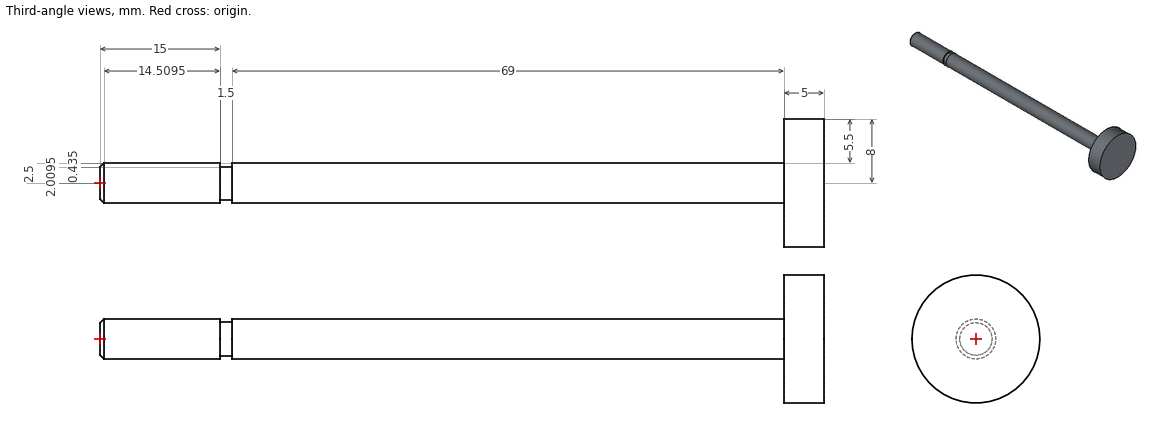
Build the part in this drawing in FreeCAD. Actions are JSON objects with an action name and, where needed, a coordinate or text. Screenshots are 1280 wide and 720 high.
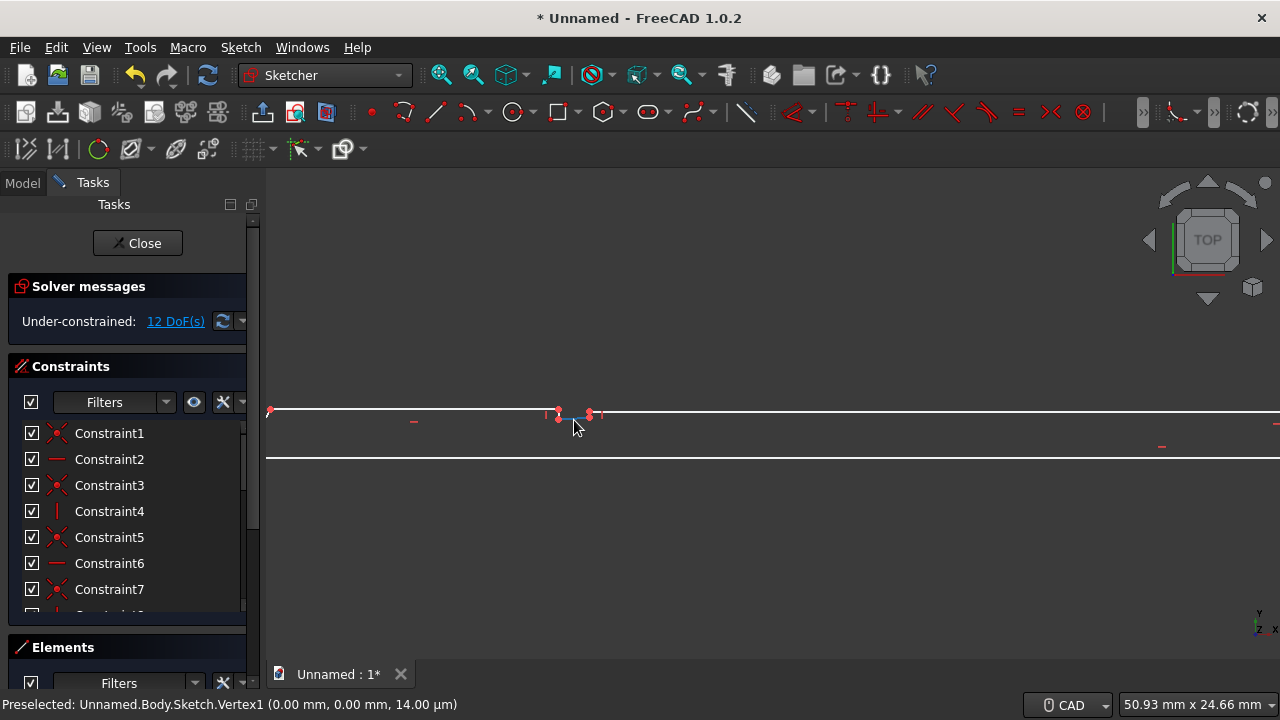
{"action": "left_click", "coordinate": [574, 419]}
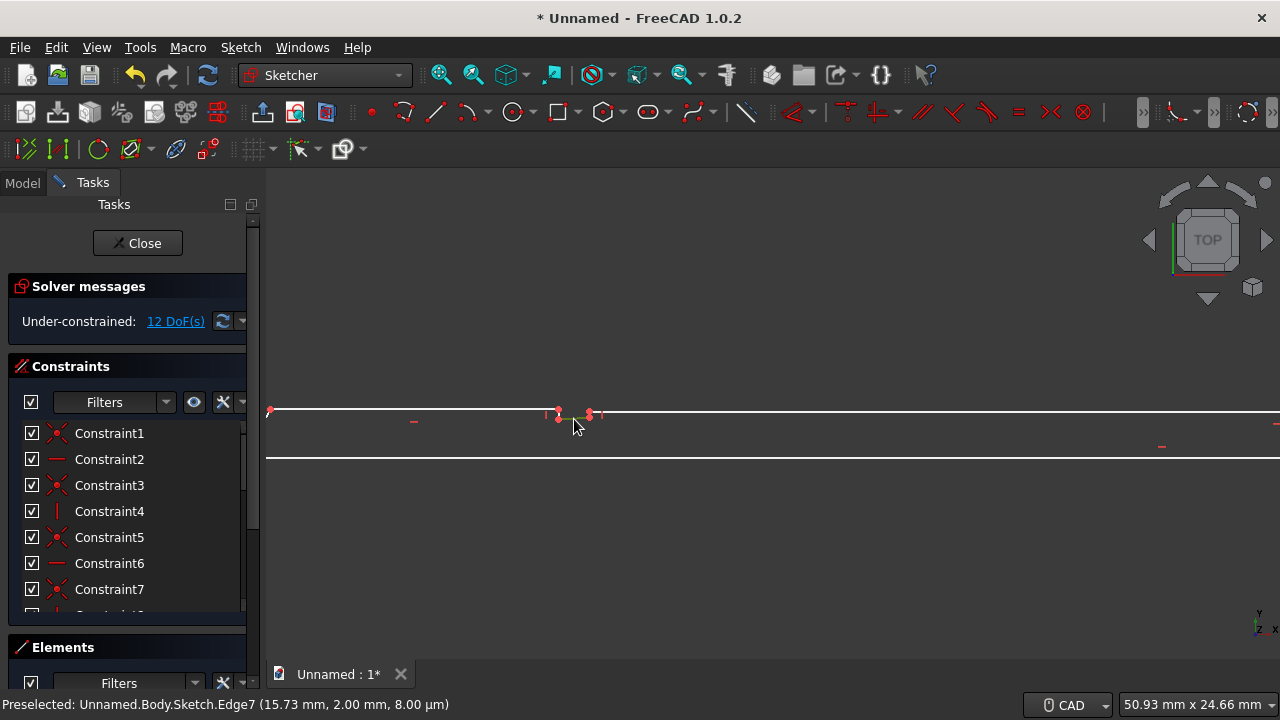
{"action": "key", "text": "h"}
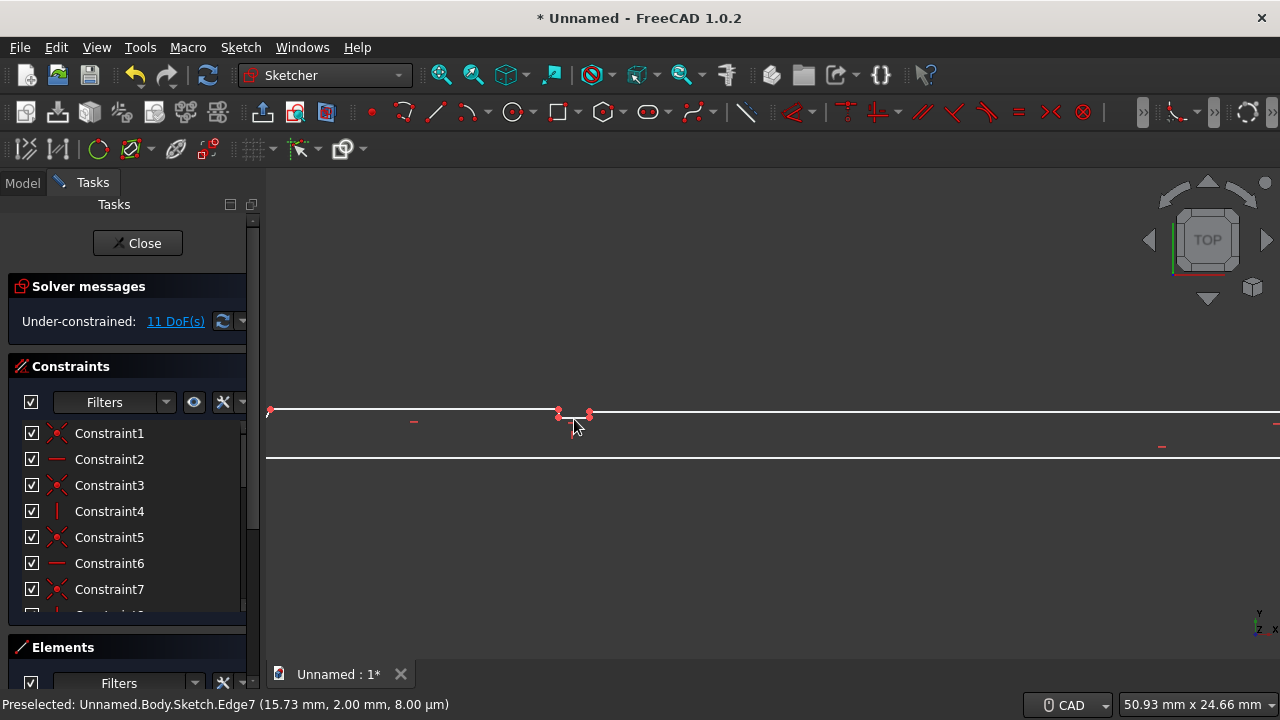
{"action": "scroll", "coordinate": [507, 428], "scroll_direction": "down", "scroll_amount": 6}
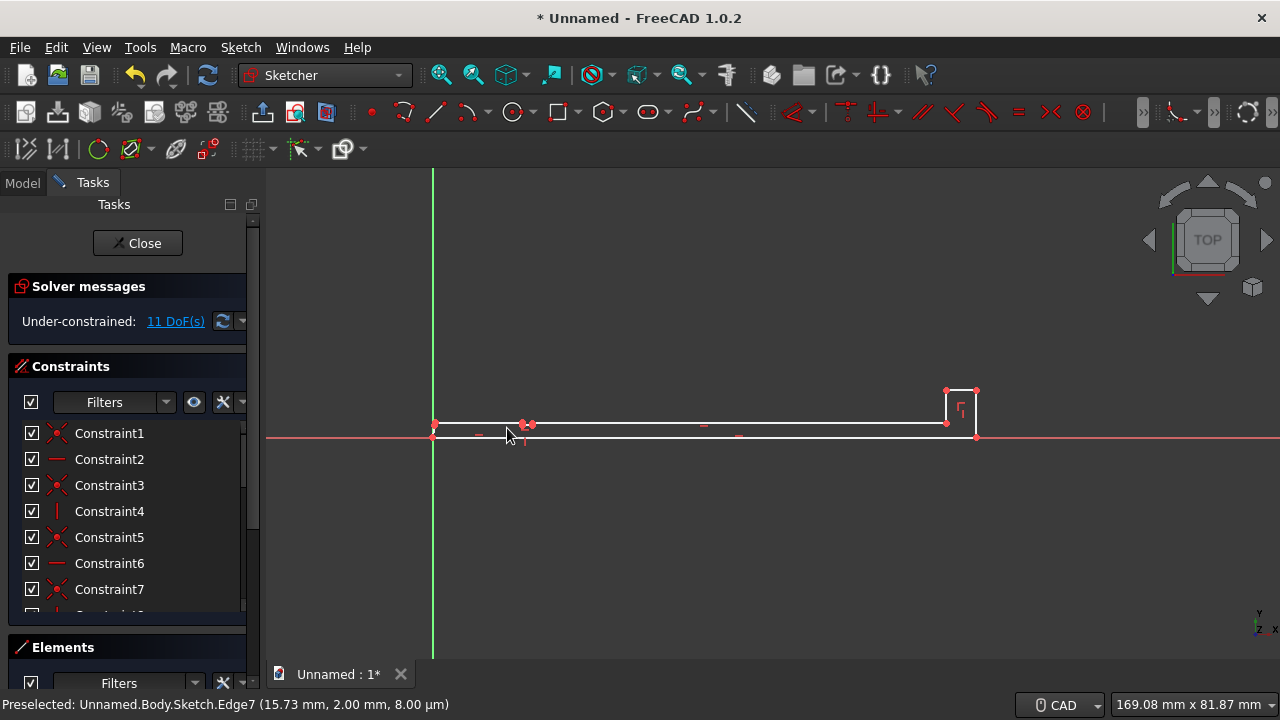
{"action": "scroll", "coordinate": [434, 429], "scroll_direction": "up", "scroll_amount": 7}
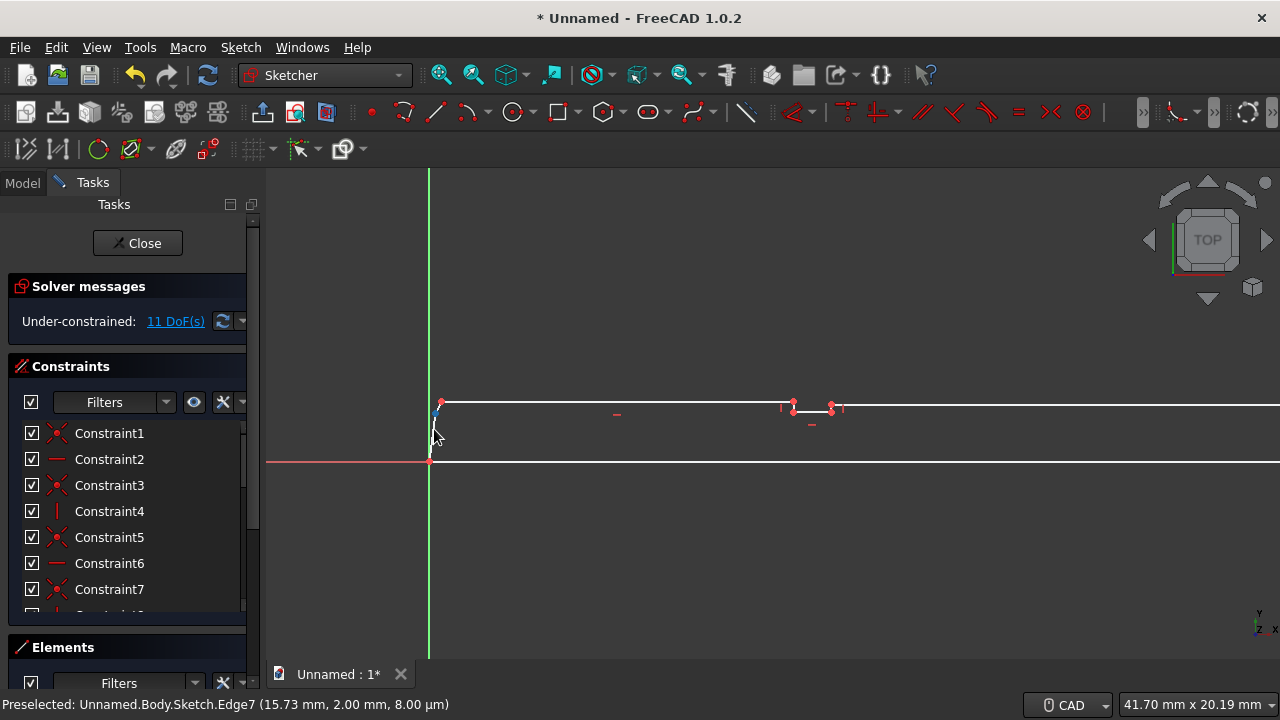
{"action": "left_click", "coordinate": [434, 428]}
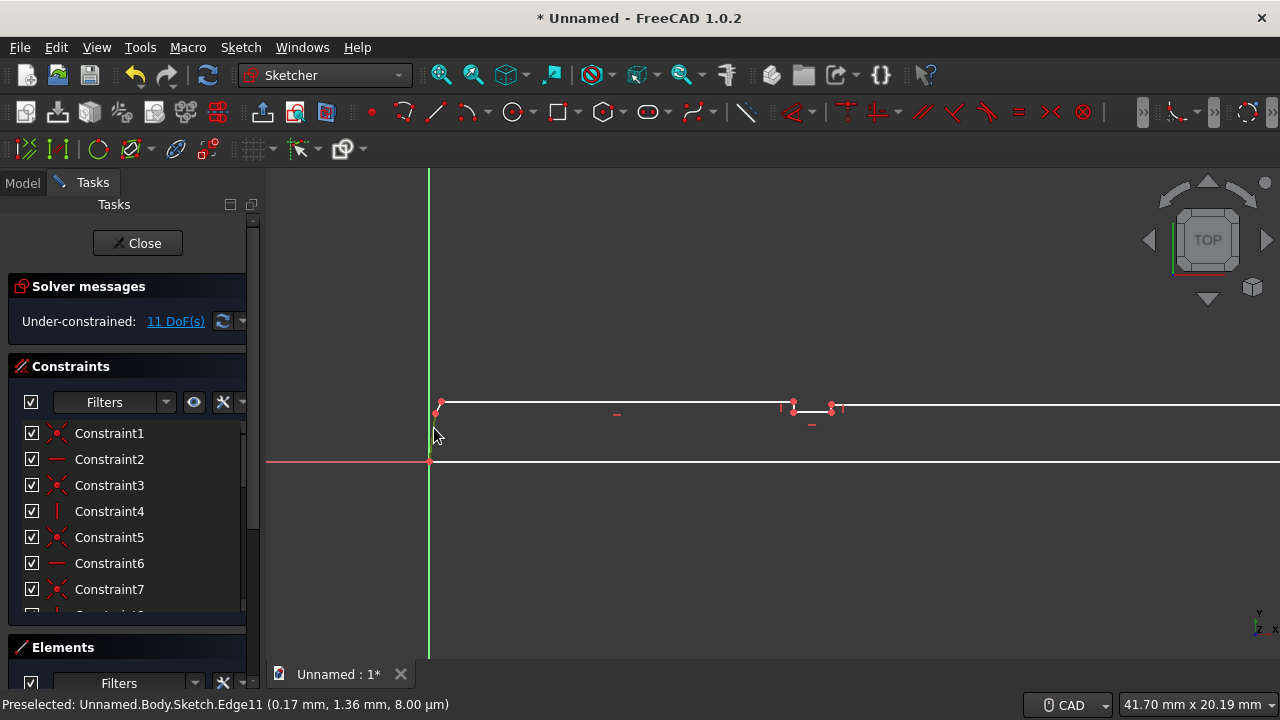
{"action": "left_click", "coordinate": [900, 112]}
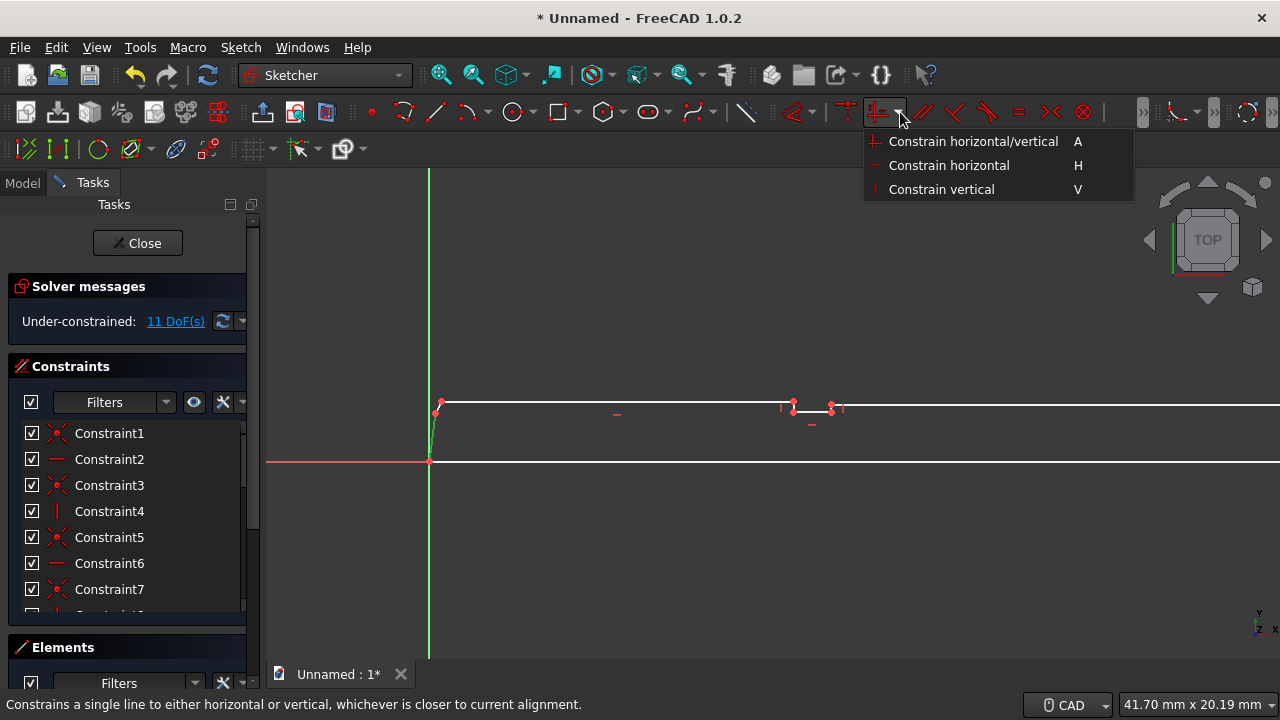
{"action": "left_click", "coordinate": [999, 189]}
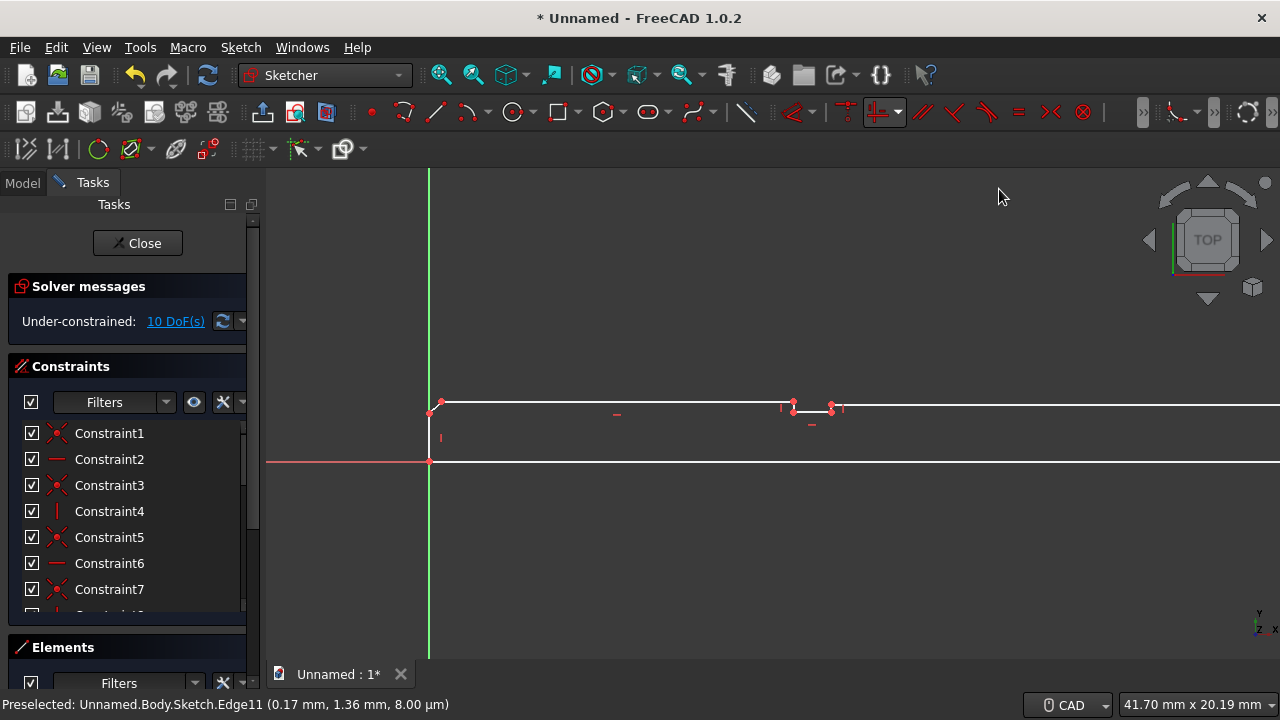
{"action": "left_click", "coordinate": [792, 112]}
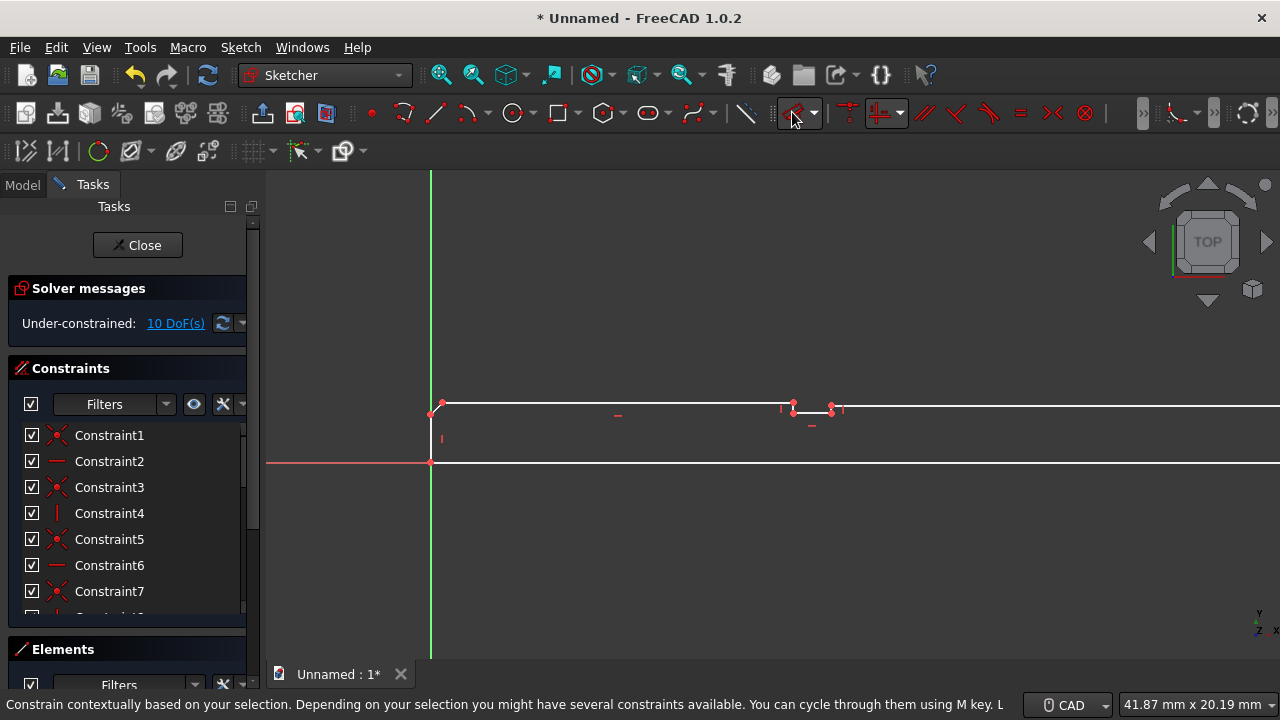
{"action": "scroll", "coordinate": [435, 430], "scroll_direction": "down", "scroll_amount": 7}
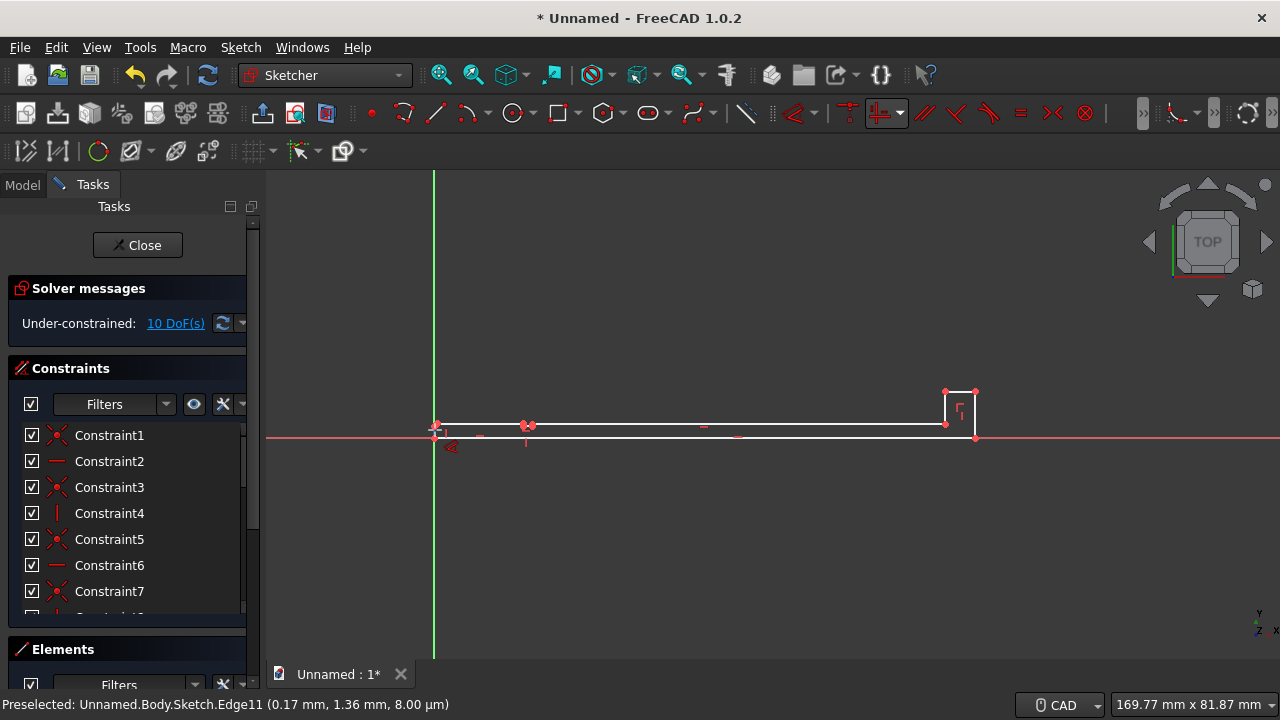
{"action": "left_click", "coordinate": [975, 424]}
{"action": "left_click", "coordinate": [1009, 415]}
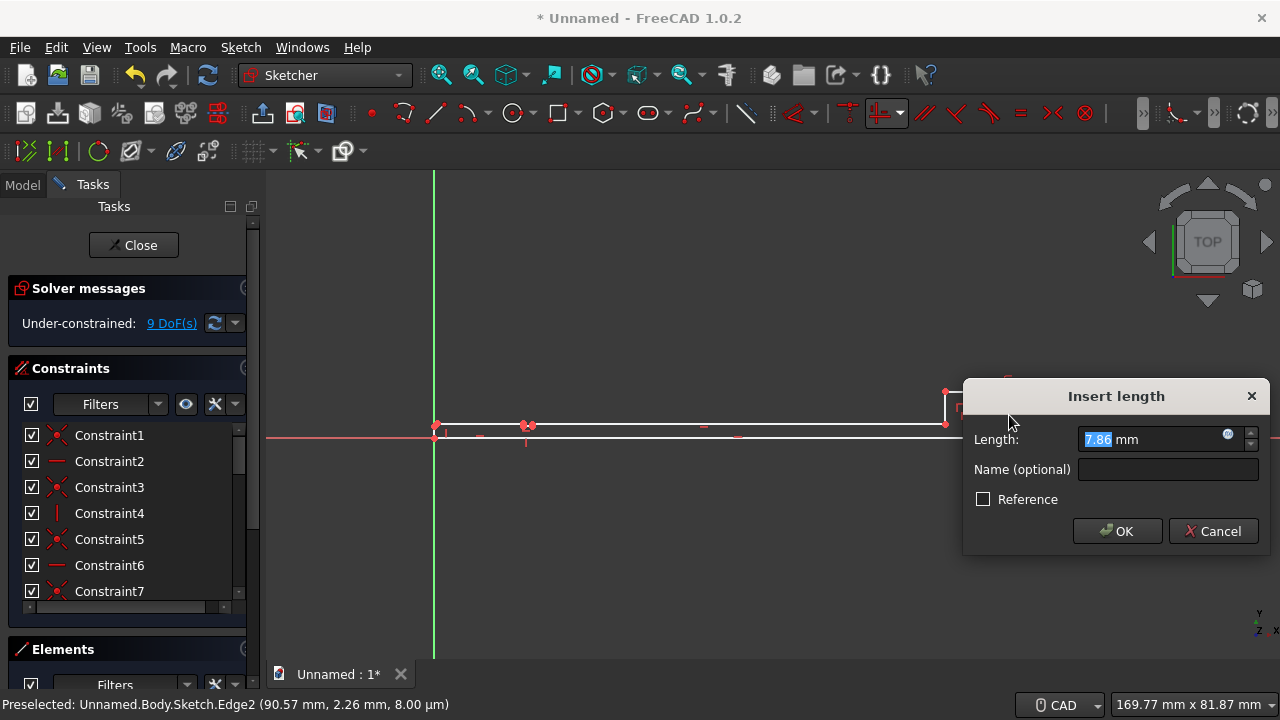
{"action": "type", "text": "8"}
{"action": "key", "text": "Return"}